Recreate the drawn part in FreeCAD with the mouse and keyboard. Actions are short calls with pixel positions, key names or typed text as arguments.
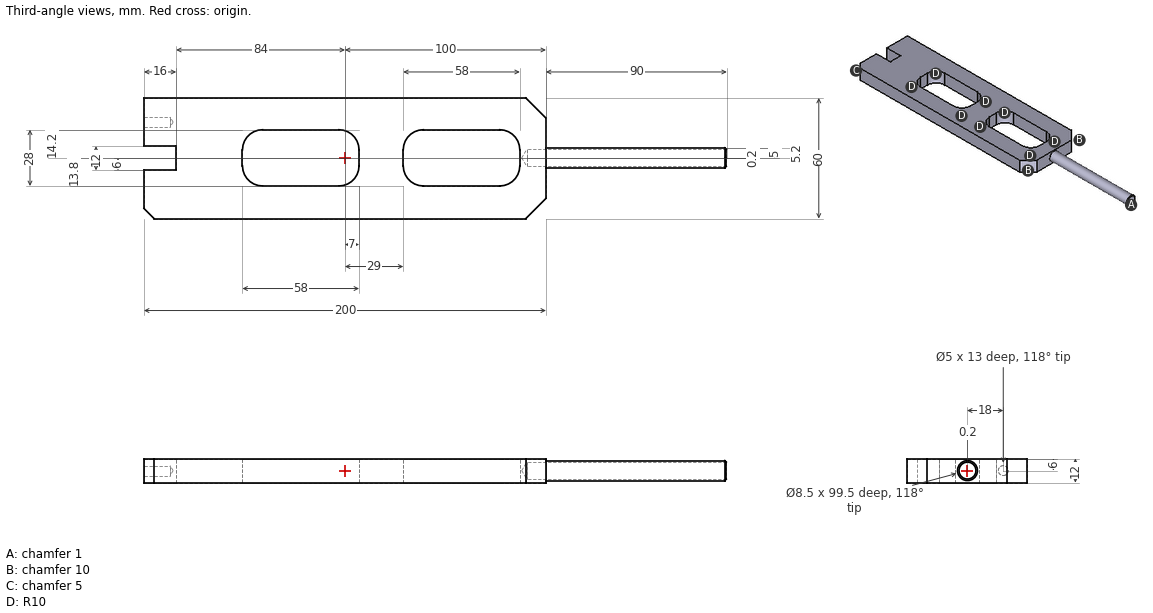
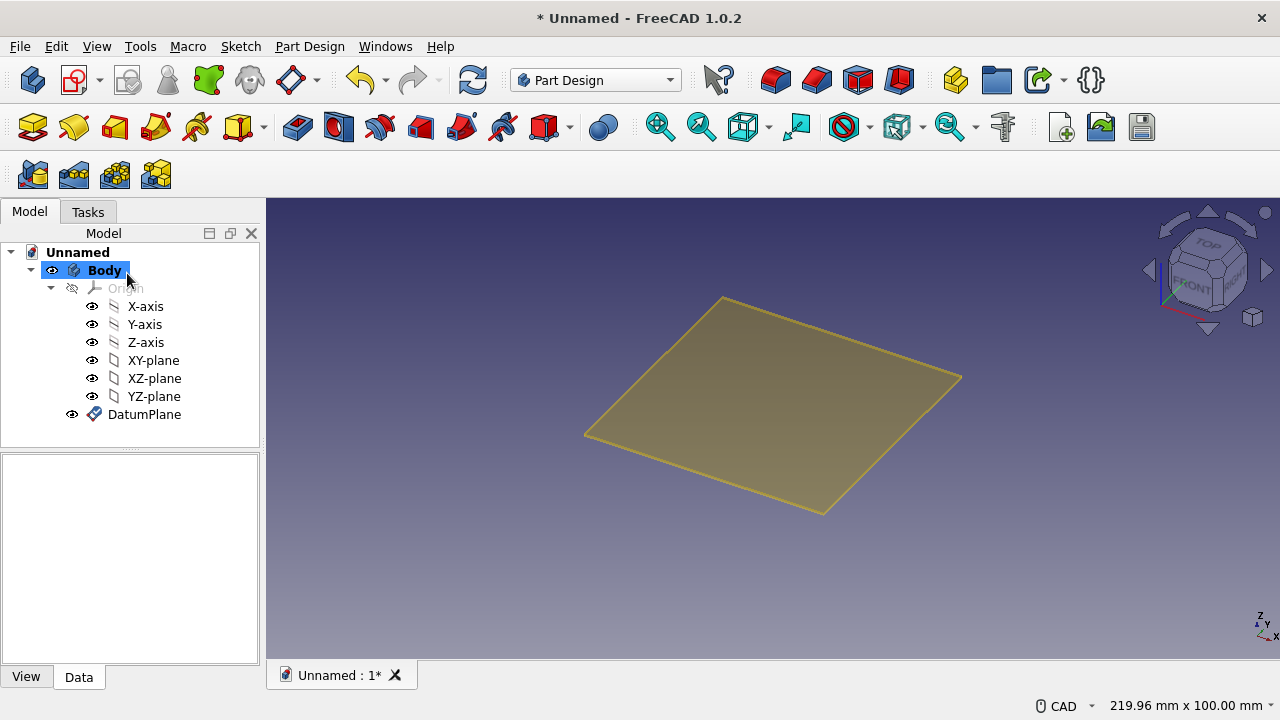
click(117, 414)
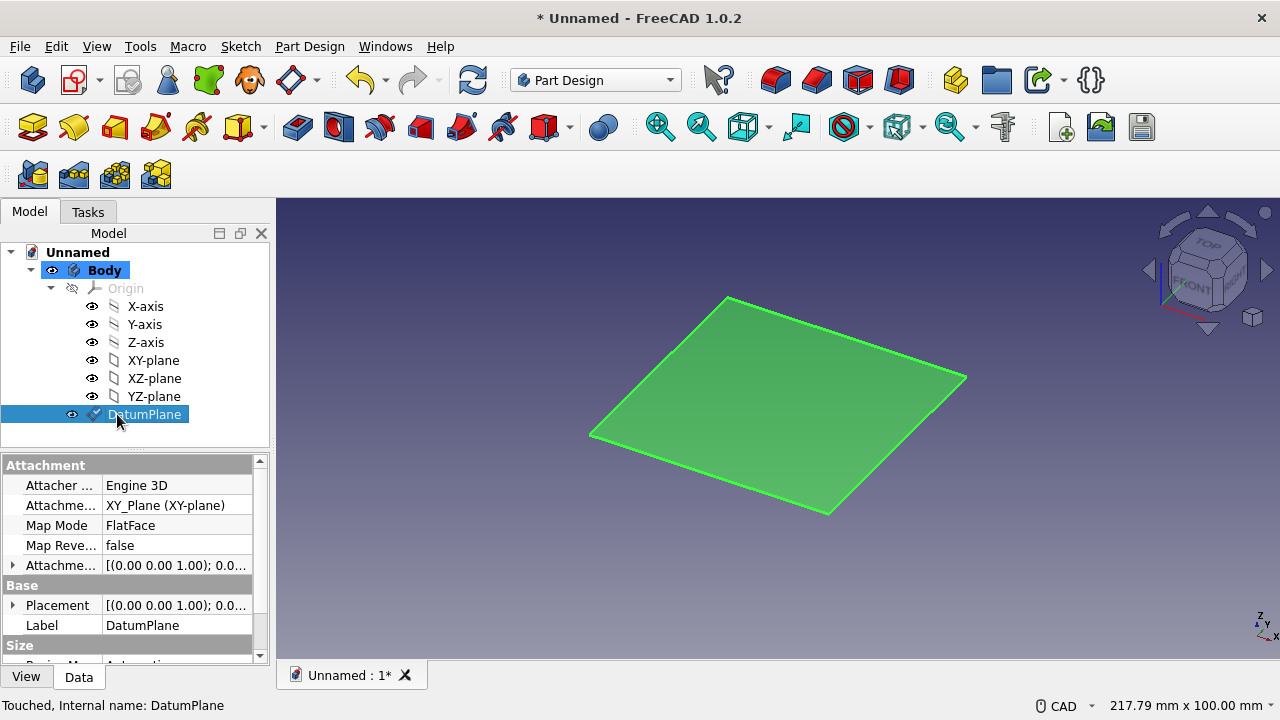
click(74, 80)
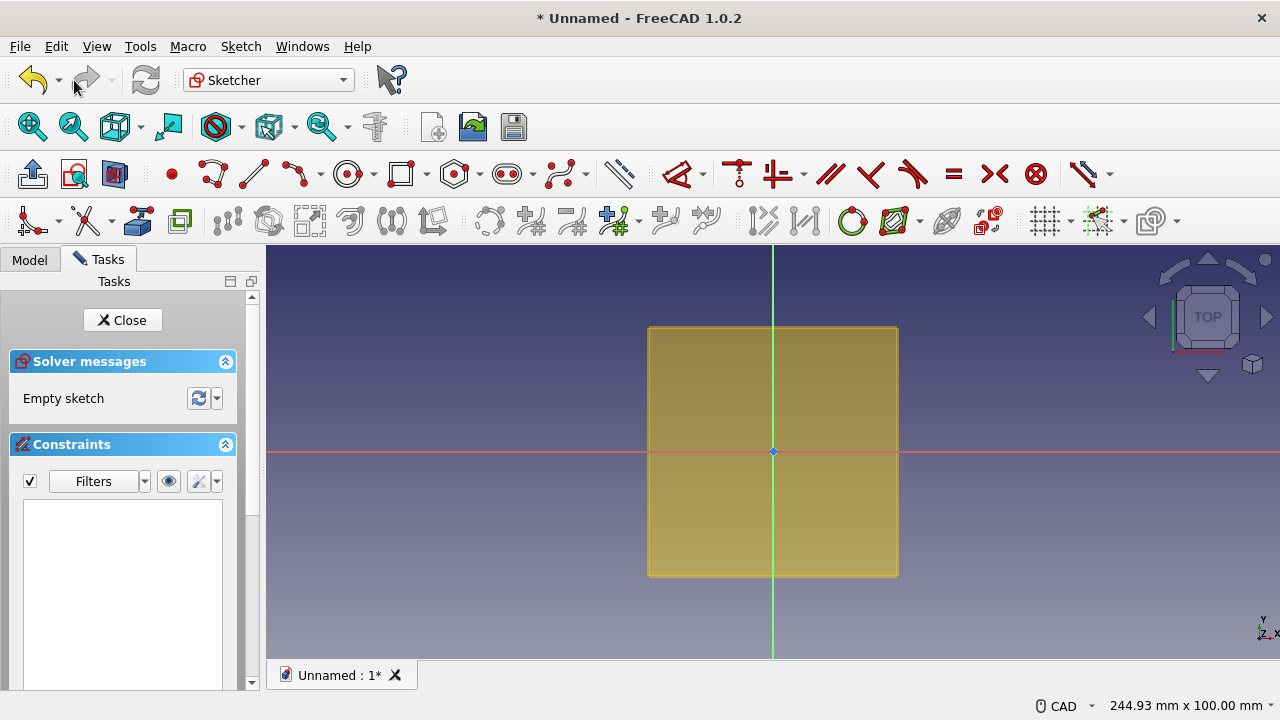
scroll(565, 452, down, 2)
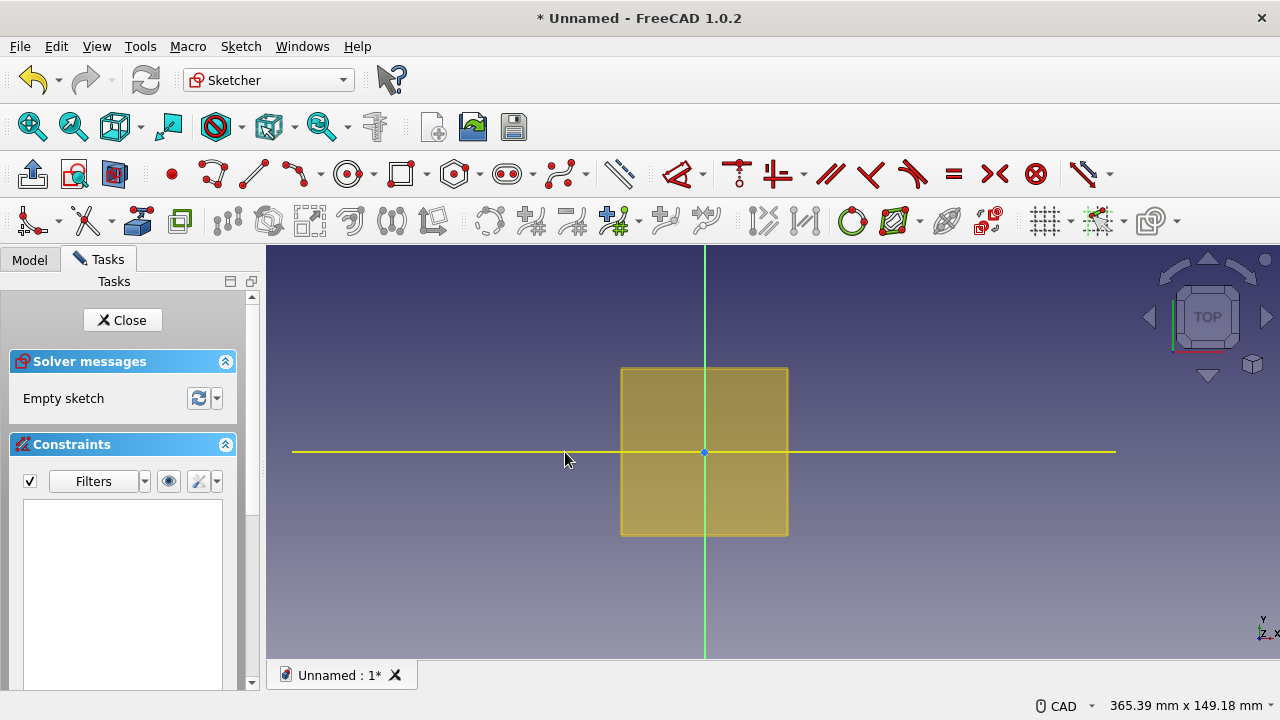
key(g)
key(v)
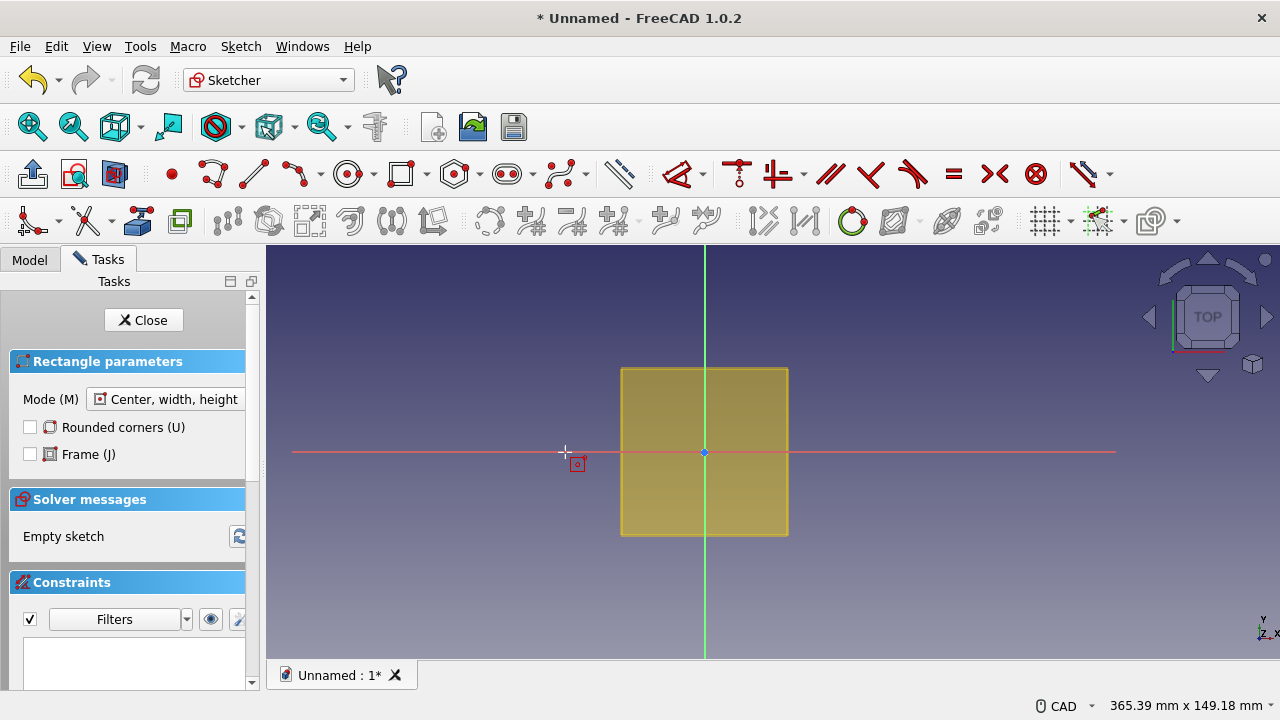
click(705, 452)
move(982, 369)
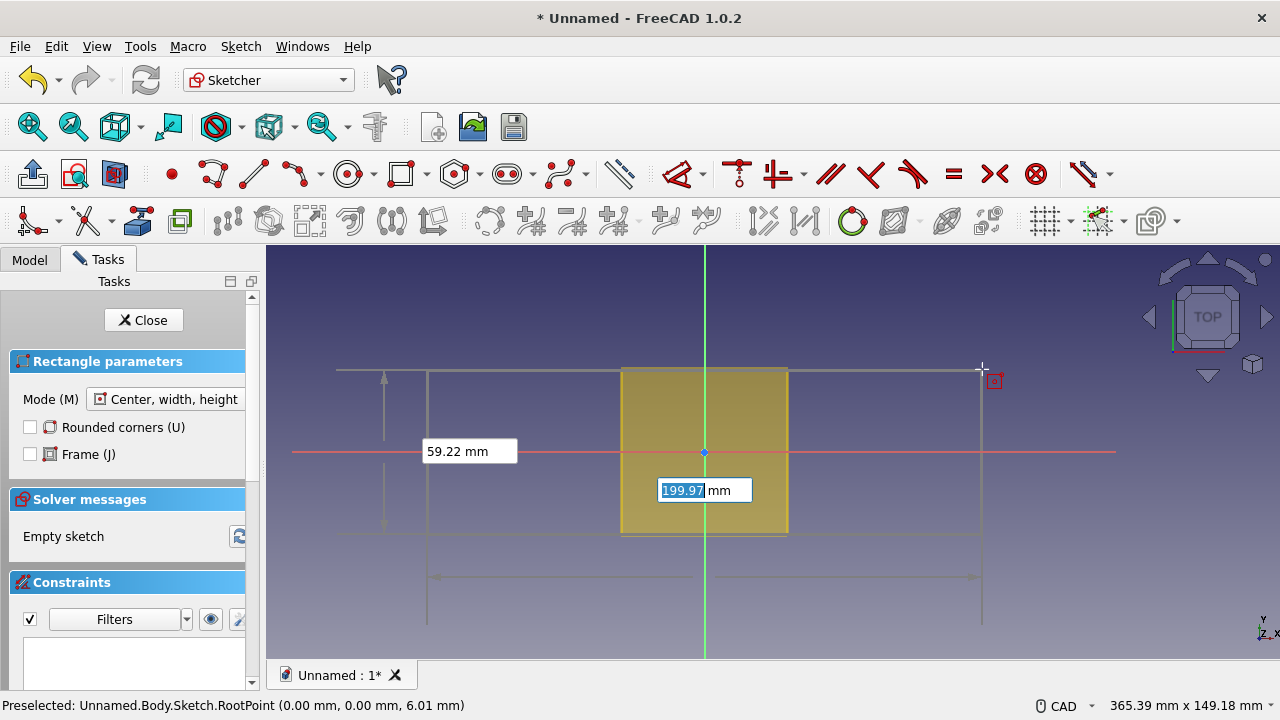
text(200)
key(Tab)
text(60)
key(Return)
key(Escape)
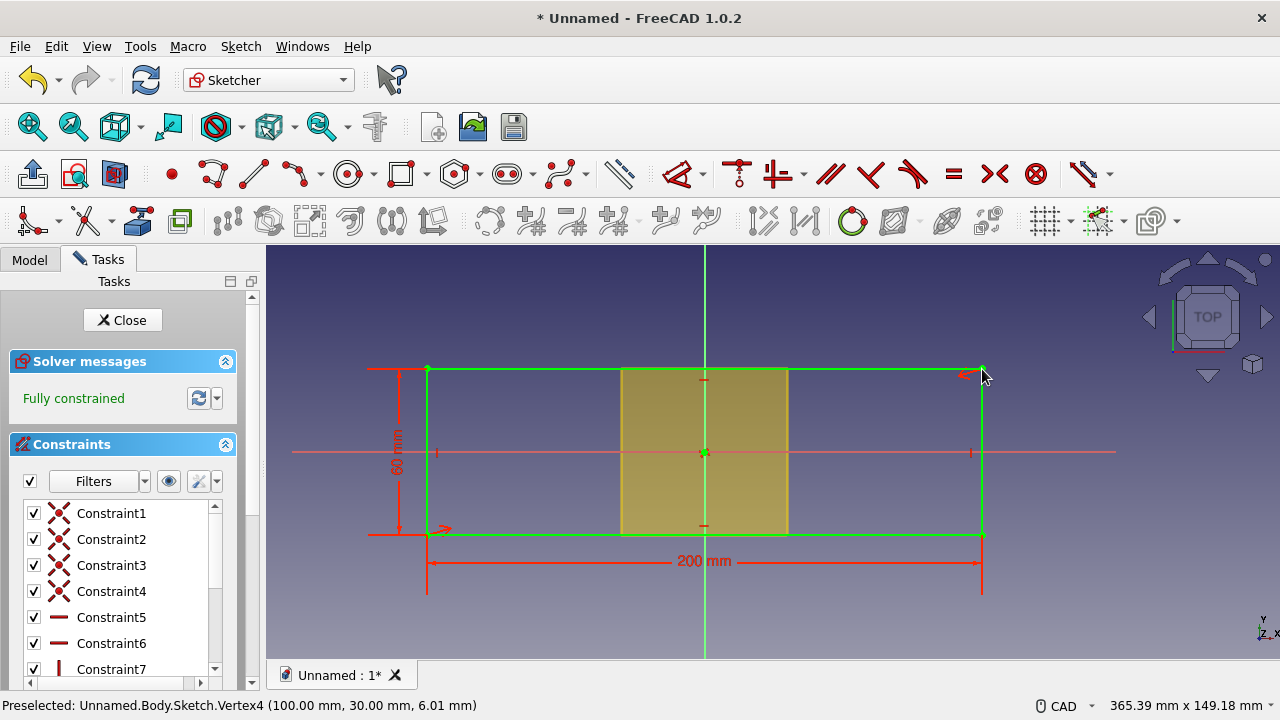
click(123, 320)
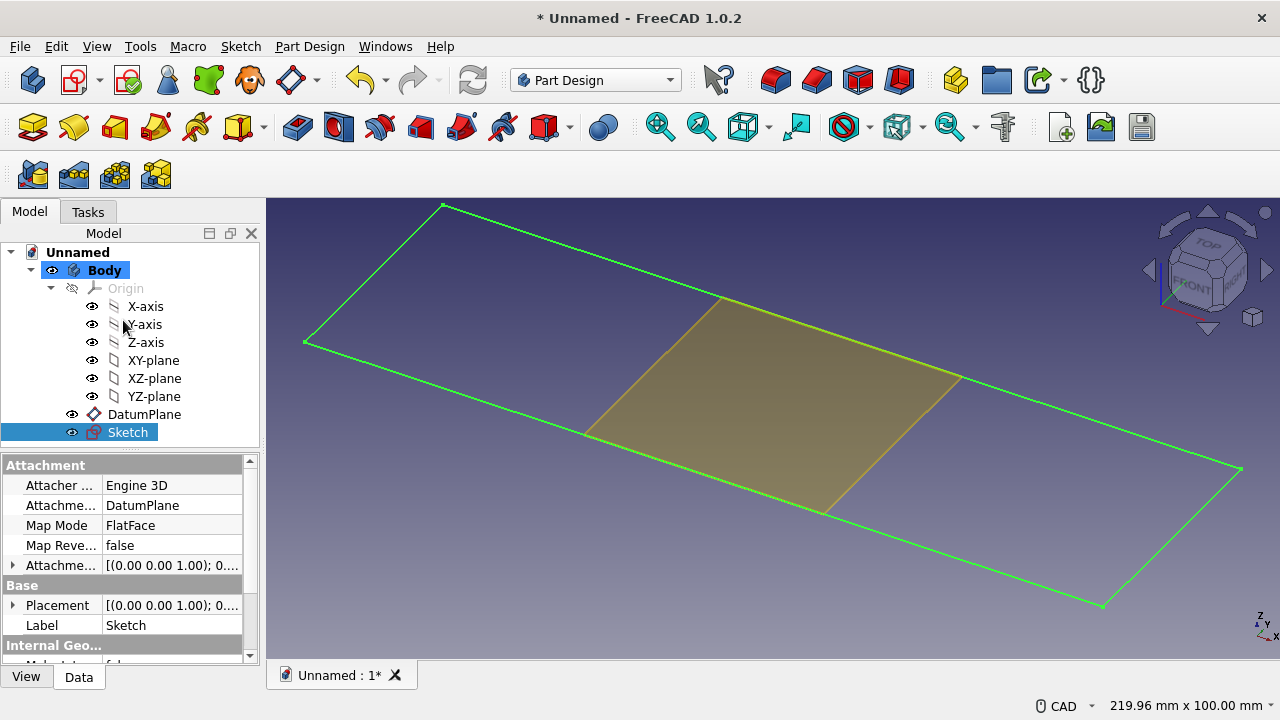
click(33, 128)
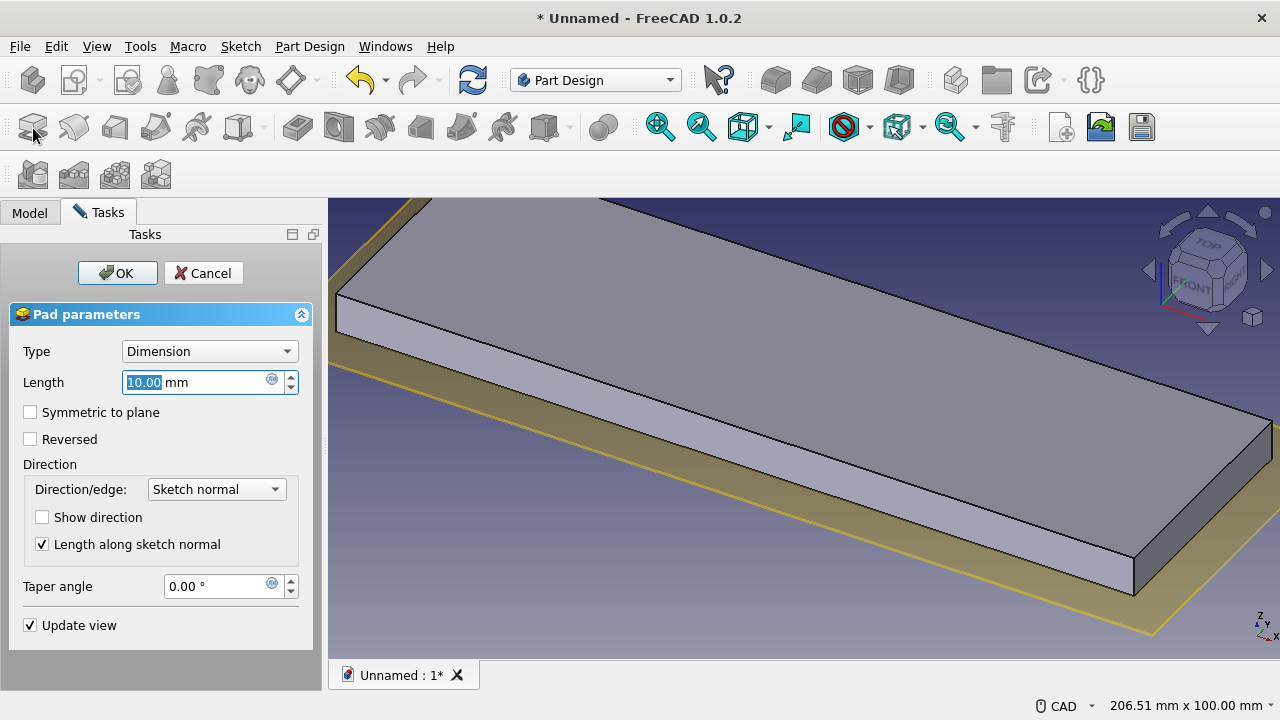
text(12)
key(Tab)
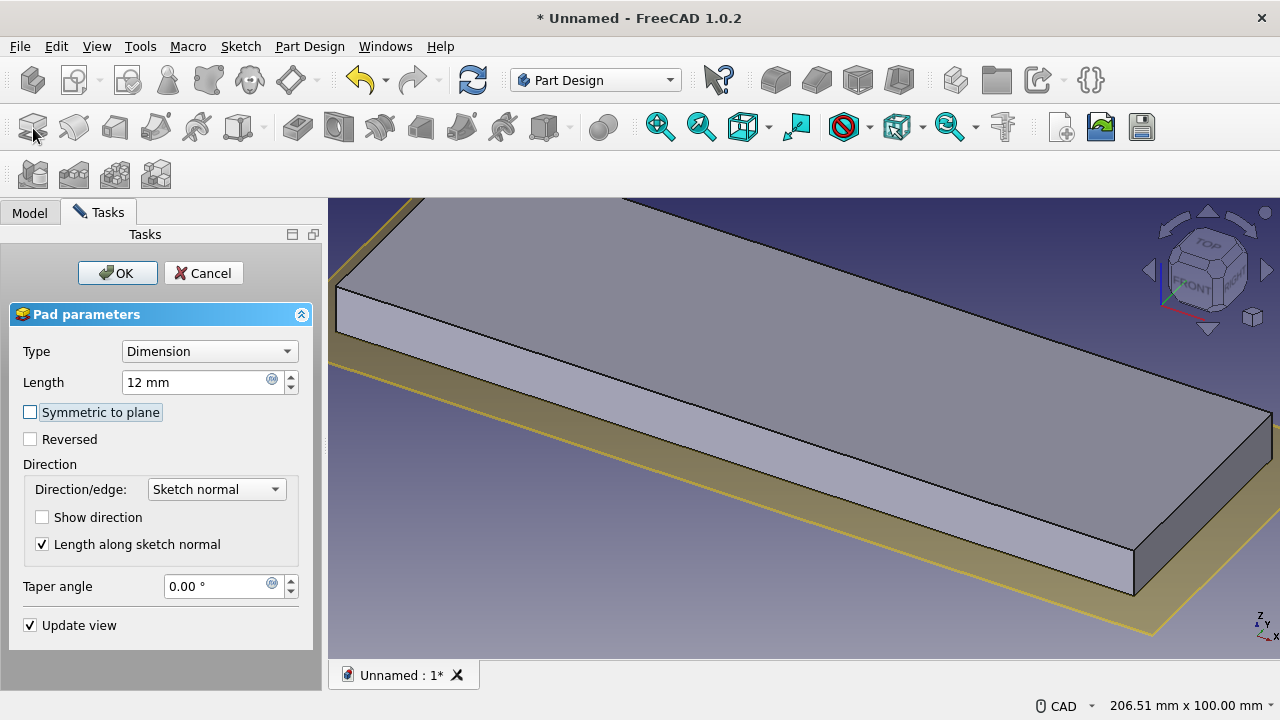
click(31, 439)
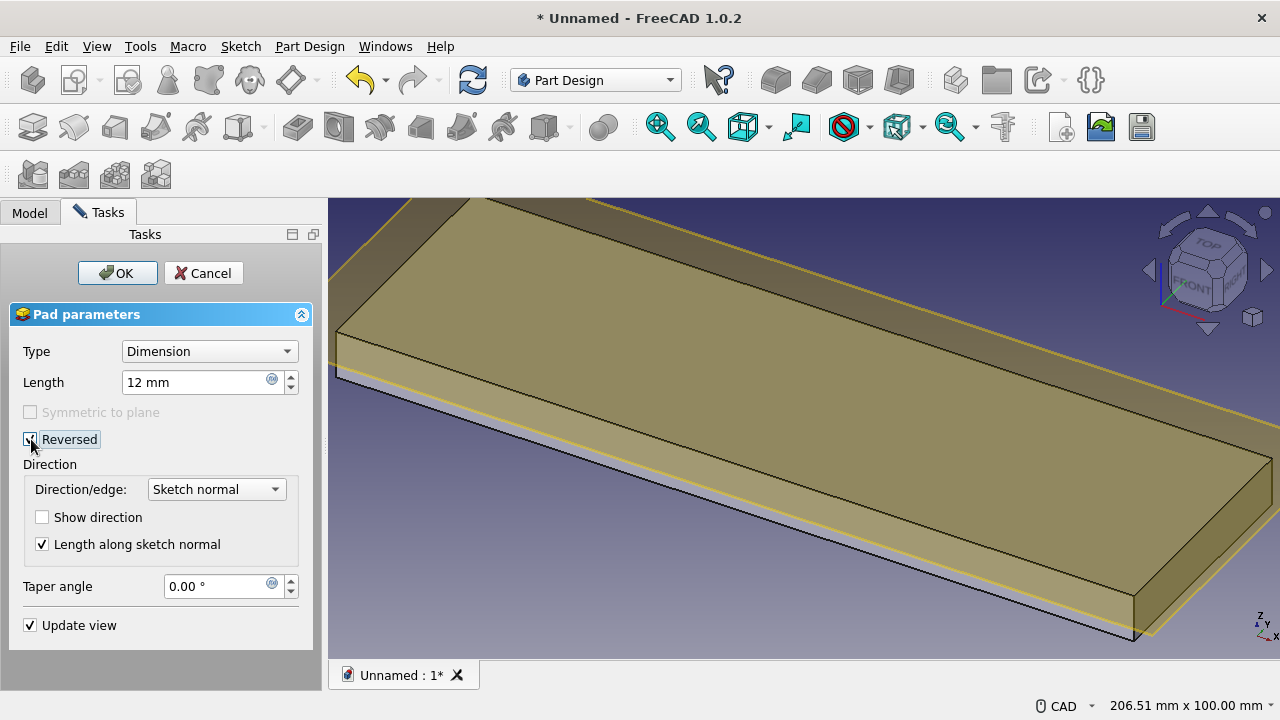
click(118, 273)